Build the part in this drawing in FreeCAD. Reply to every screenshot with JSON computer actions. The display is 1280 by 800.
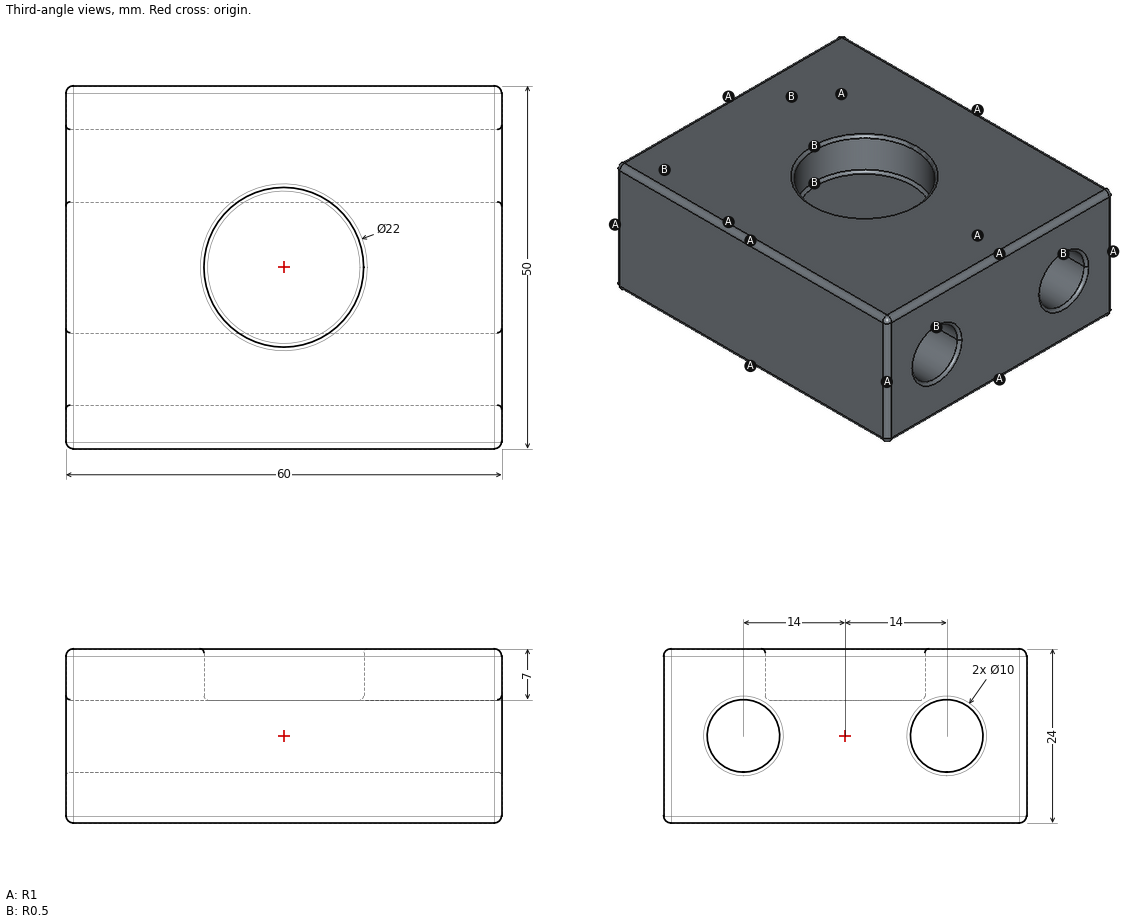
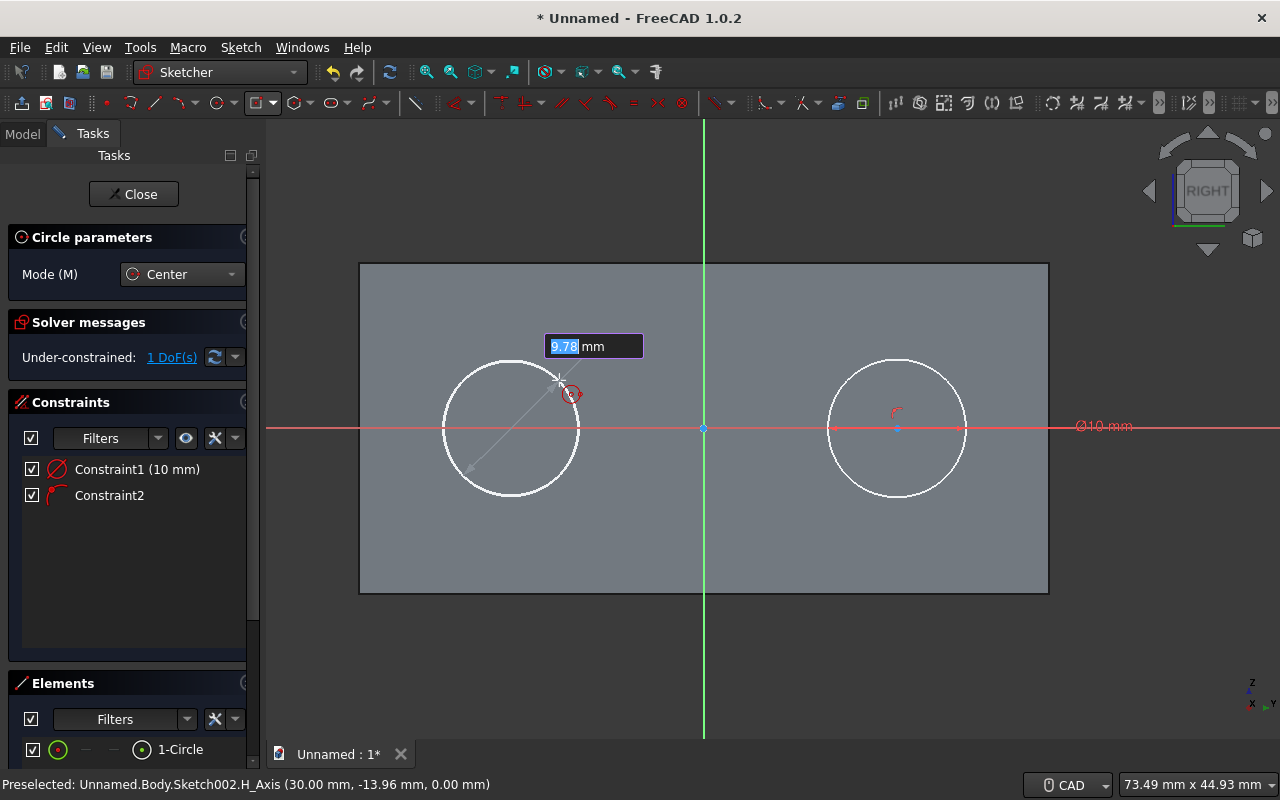
{"action": "type", "text": "10"}
{"action": "key", "text": "Return"}
{"action": "key", "text": "Escape"}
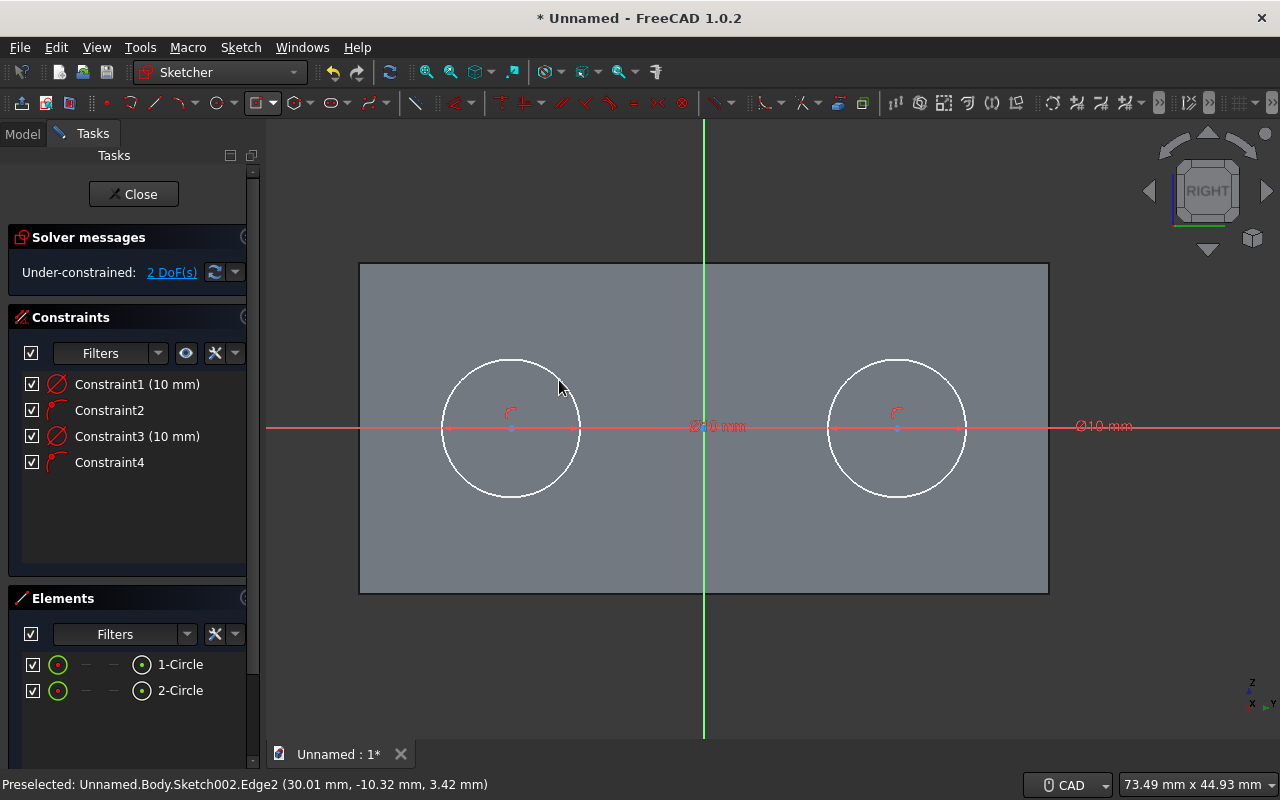
{"action": "left_click", "coordinate": [897, 428]}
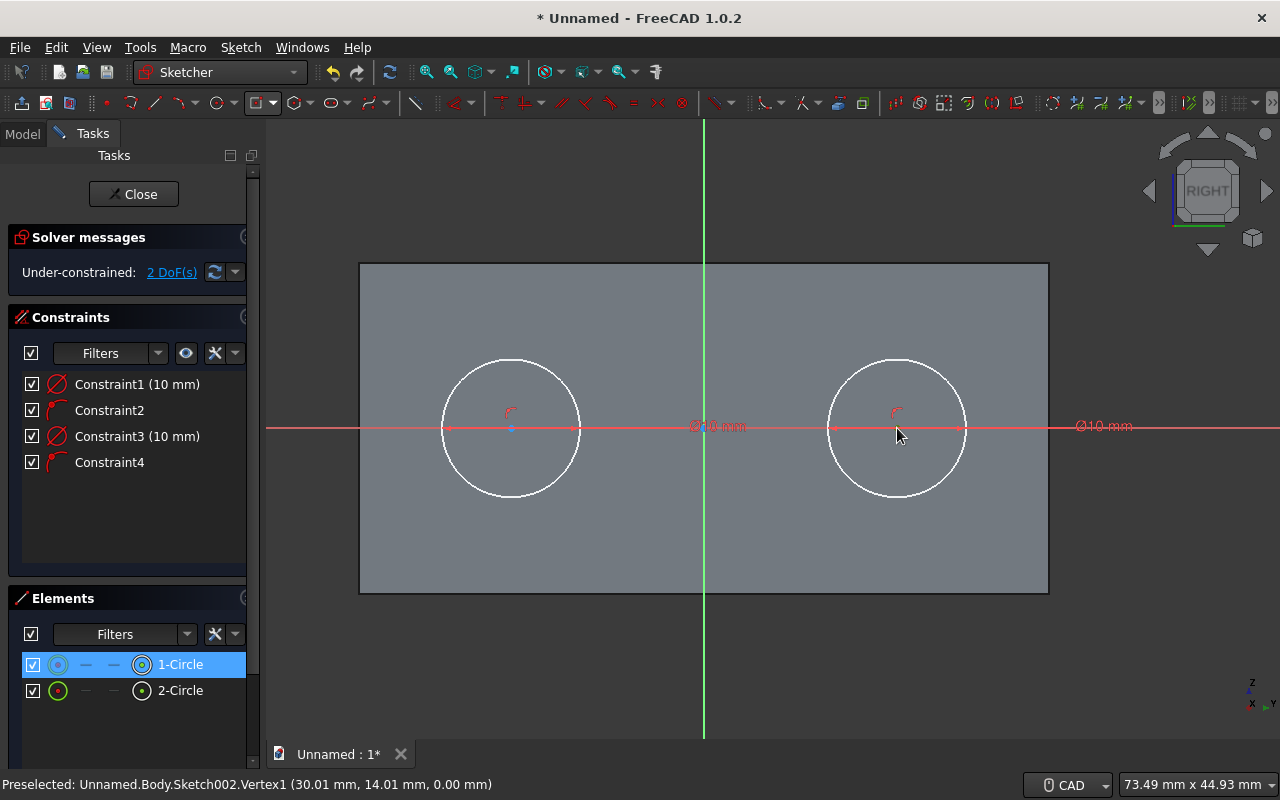
{"action": "left_click", "coordinate": [474, 104]}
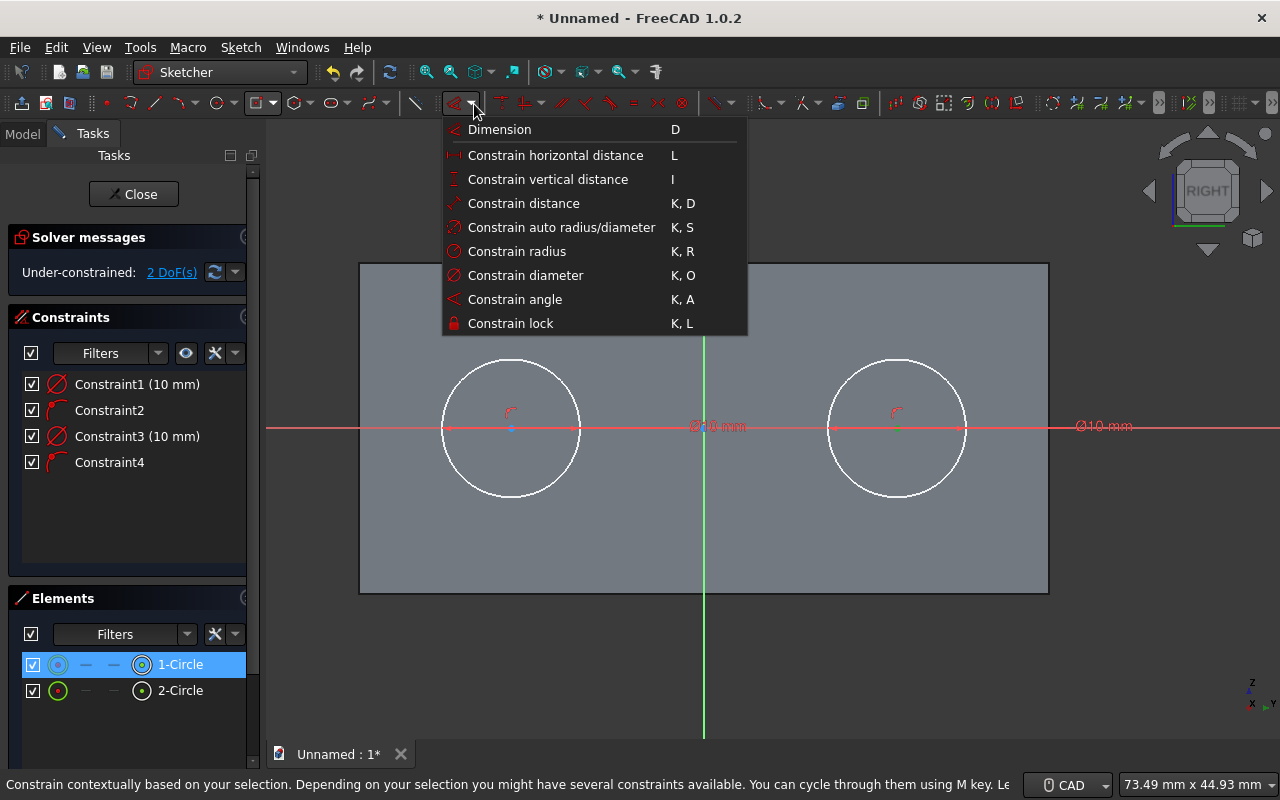
{"action": "left_click", "coordinate": [595, 155]}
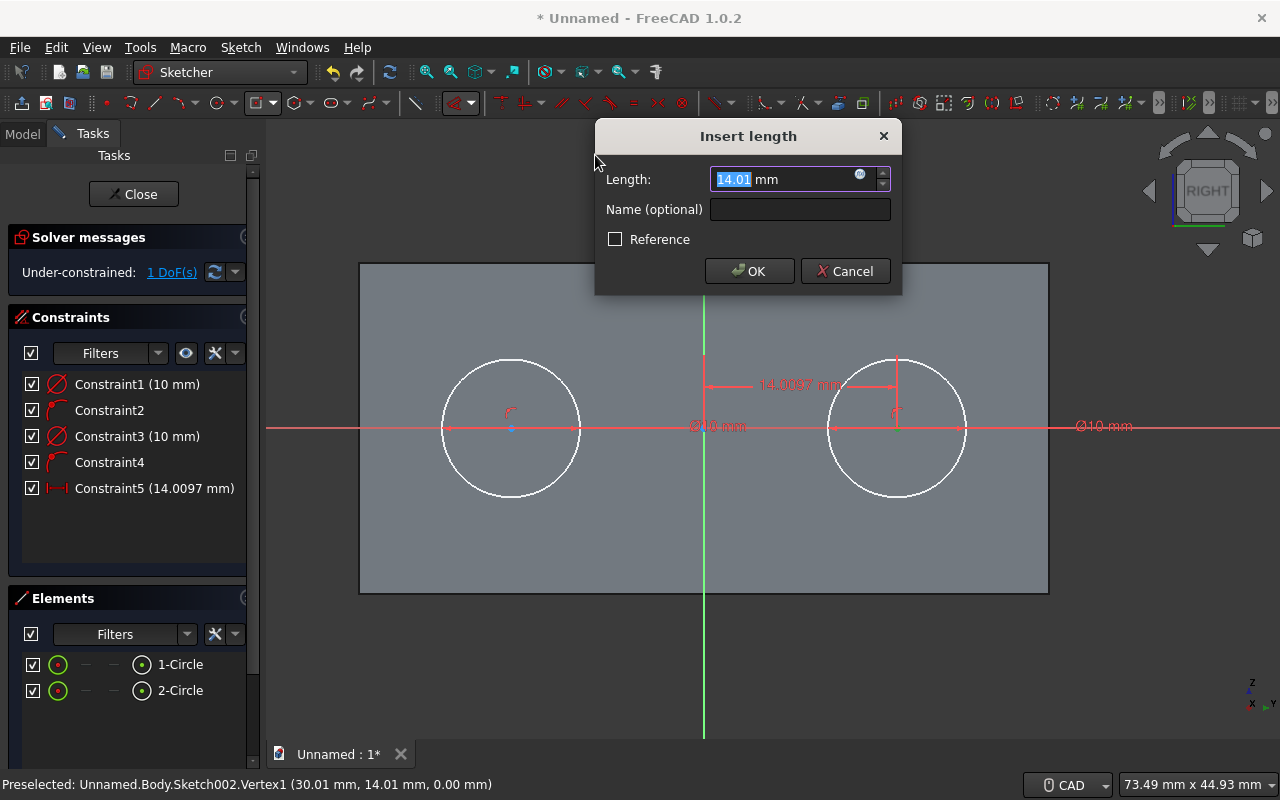
{"action": "type", "text": "14"}
{"action": "key", "text": "Return"}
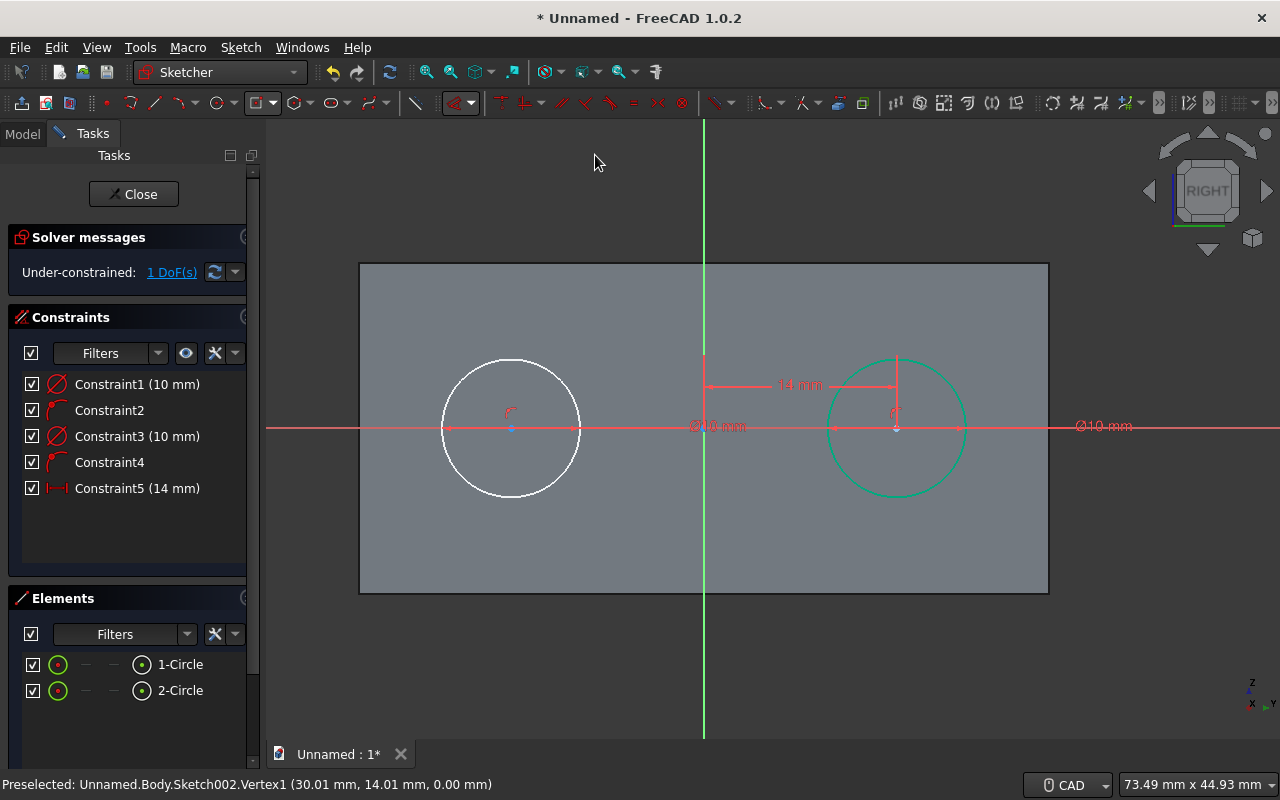
{"action": "left_click", "coordinate": [511, 428]}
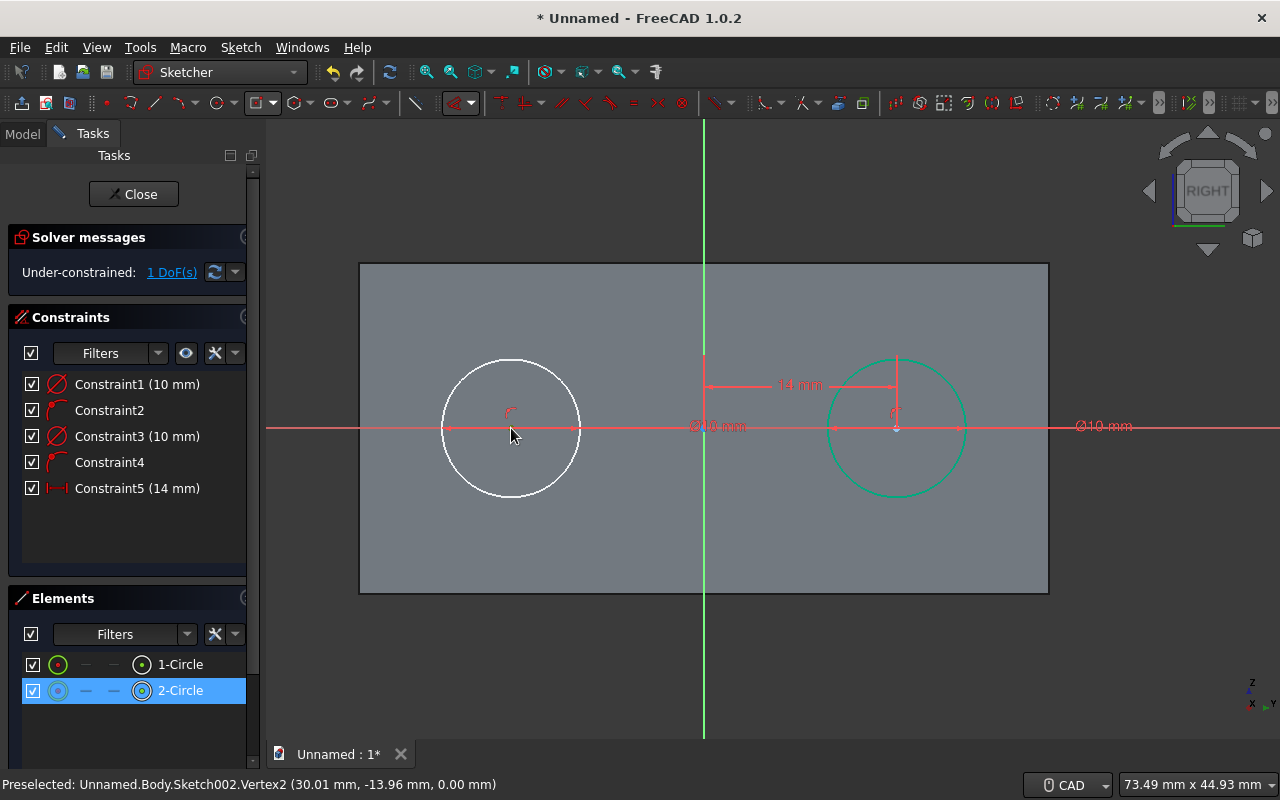
{"action": "left_click", "coordinate": [474, 104]}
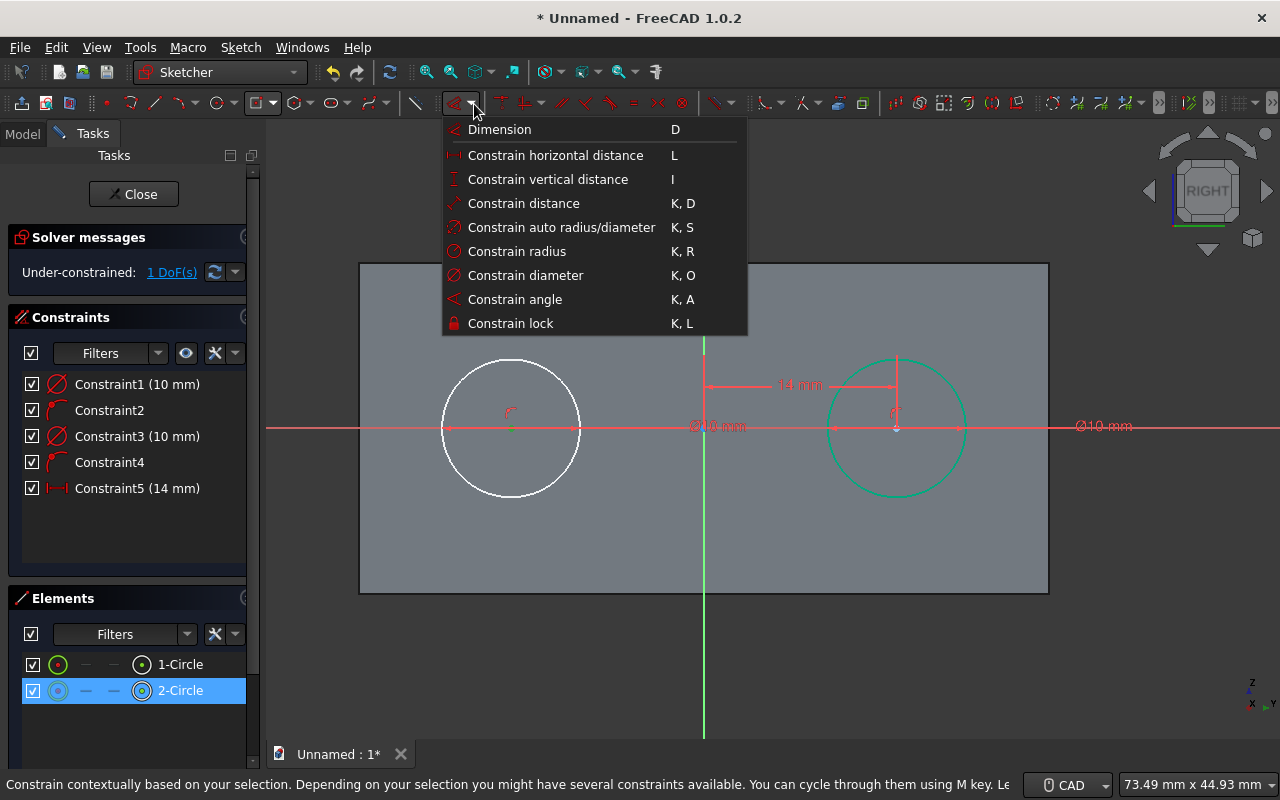
{"action": "left_click", "coordinate": [595, 155]}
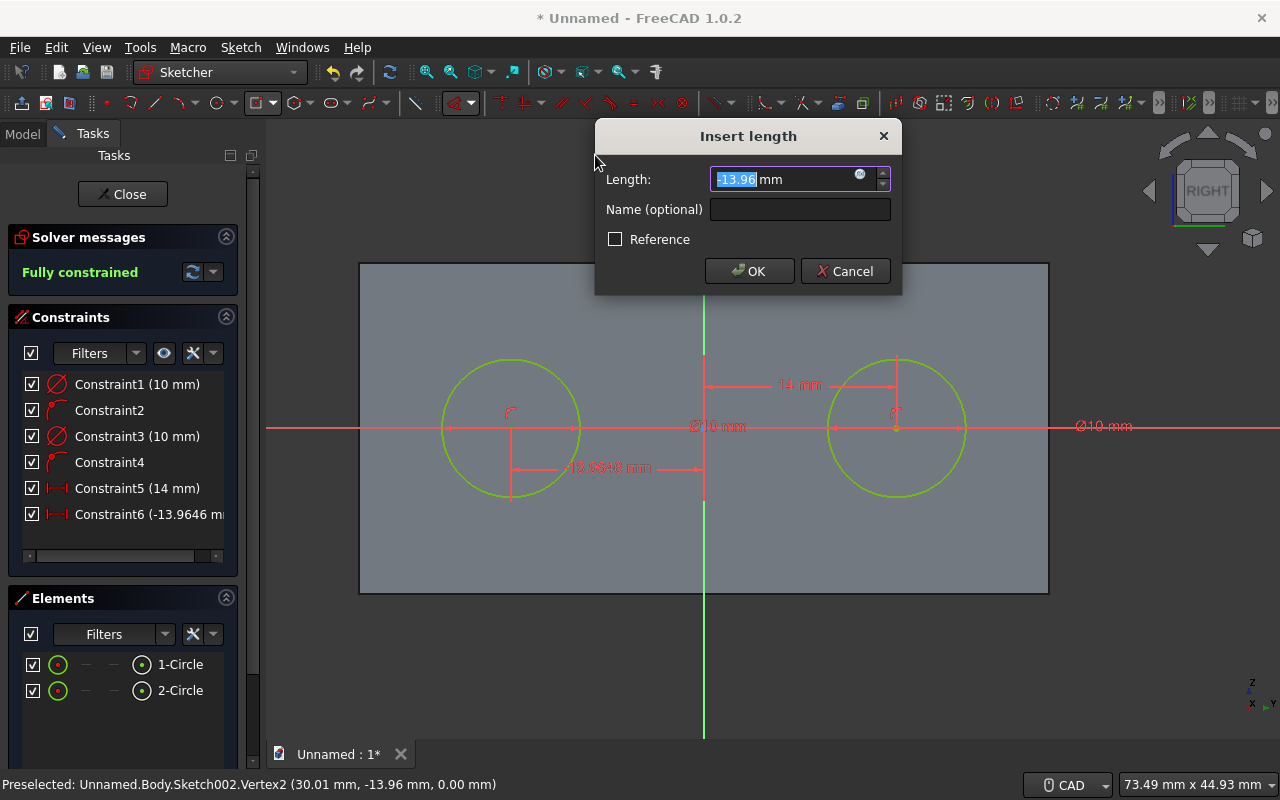
{"action": "type", "text": "-14"}
{"action": "key", "text": "Return"}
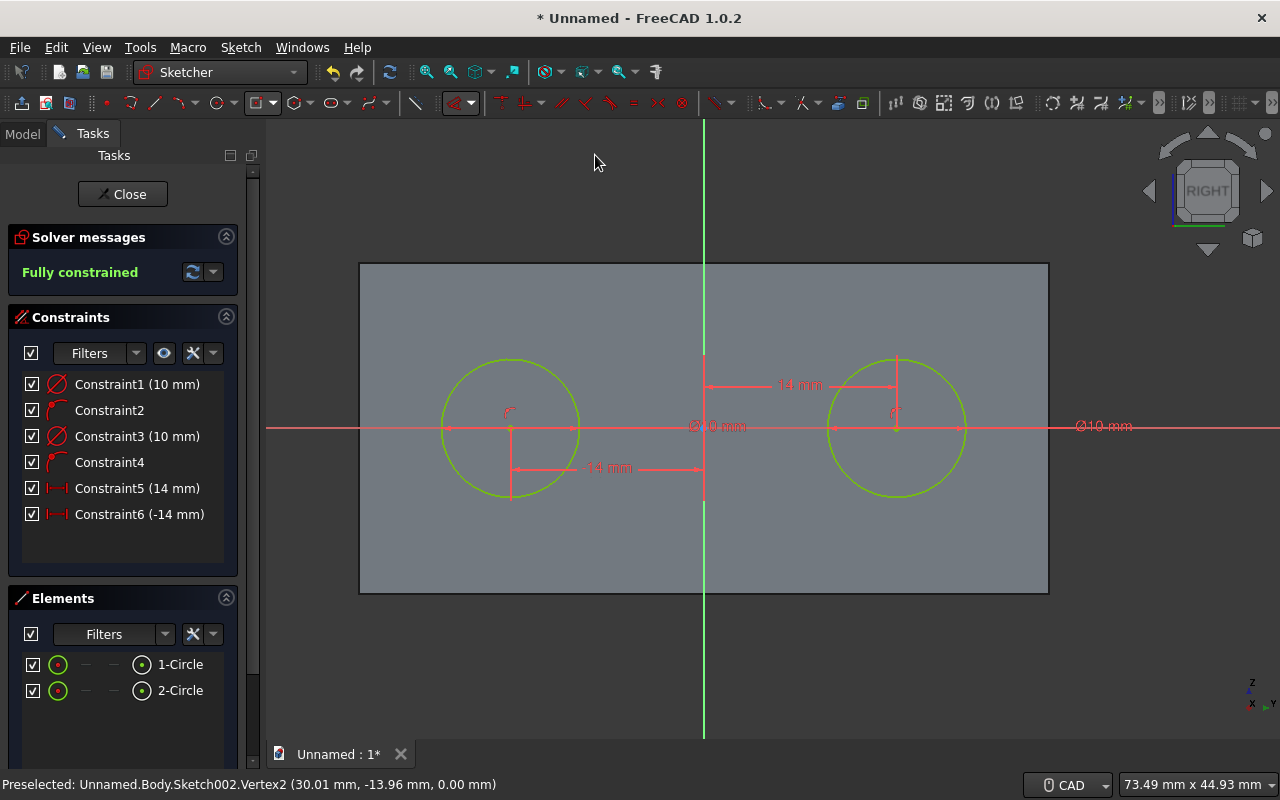
{"action": "left_click", "coordinate": [123, 194]}